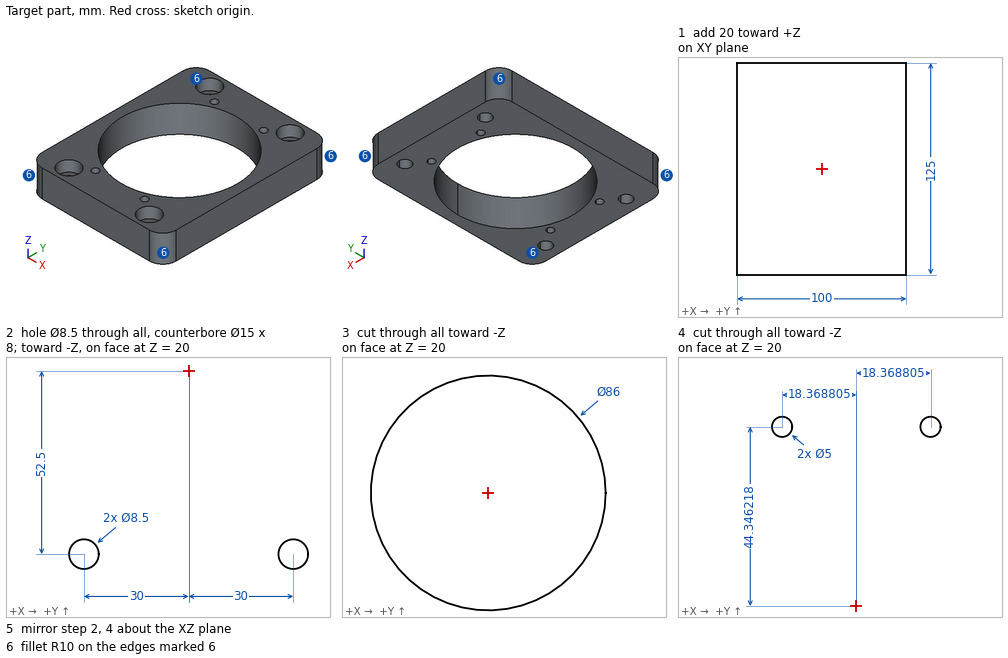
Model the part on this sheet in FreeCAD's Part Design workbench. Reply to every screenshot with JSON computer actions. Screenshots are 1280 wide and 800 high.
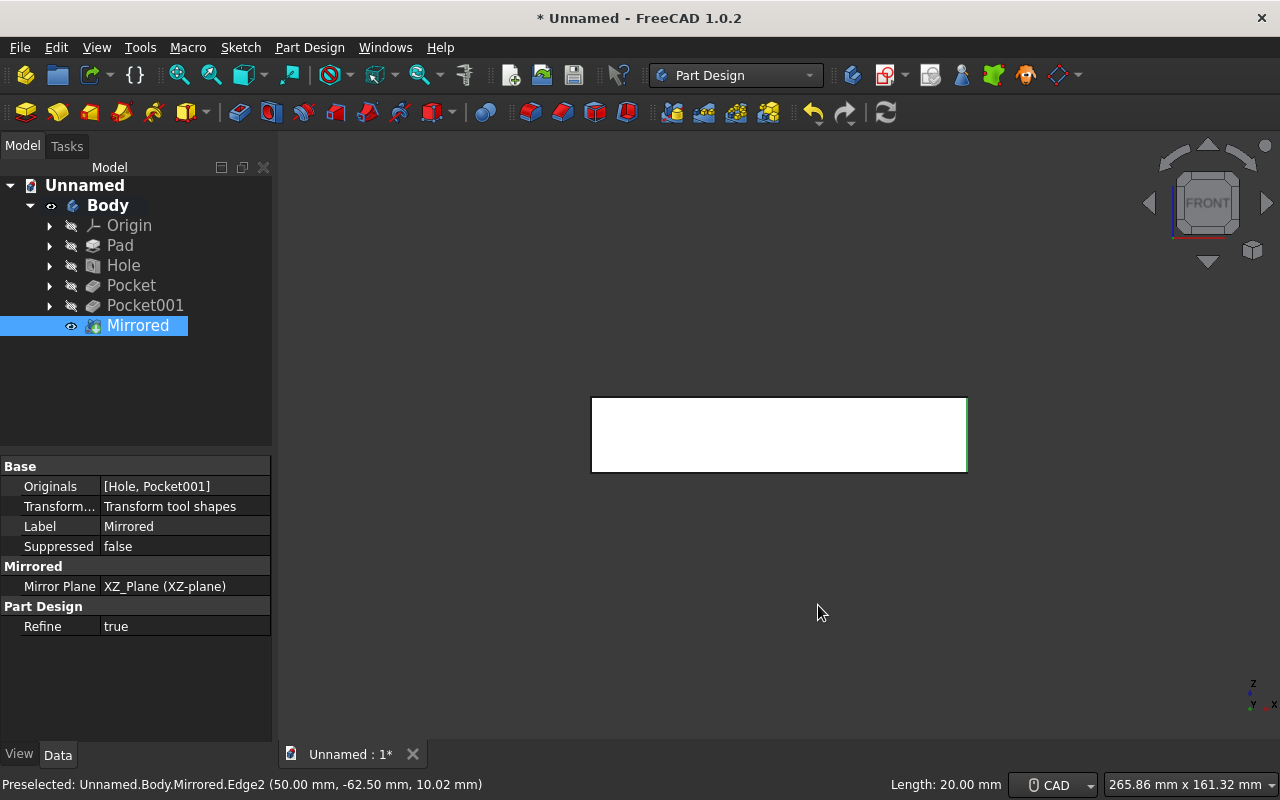
{"action": "left_click", "coordinate": [180, 76]}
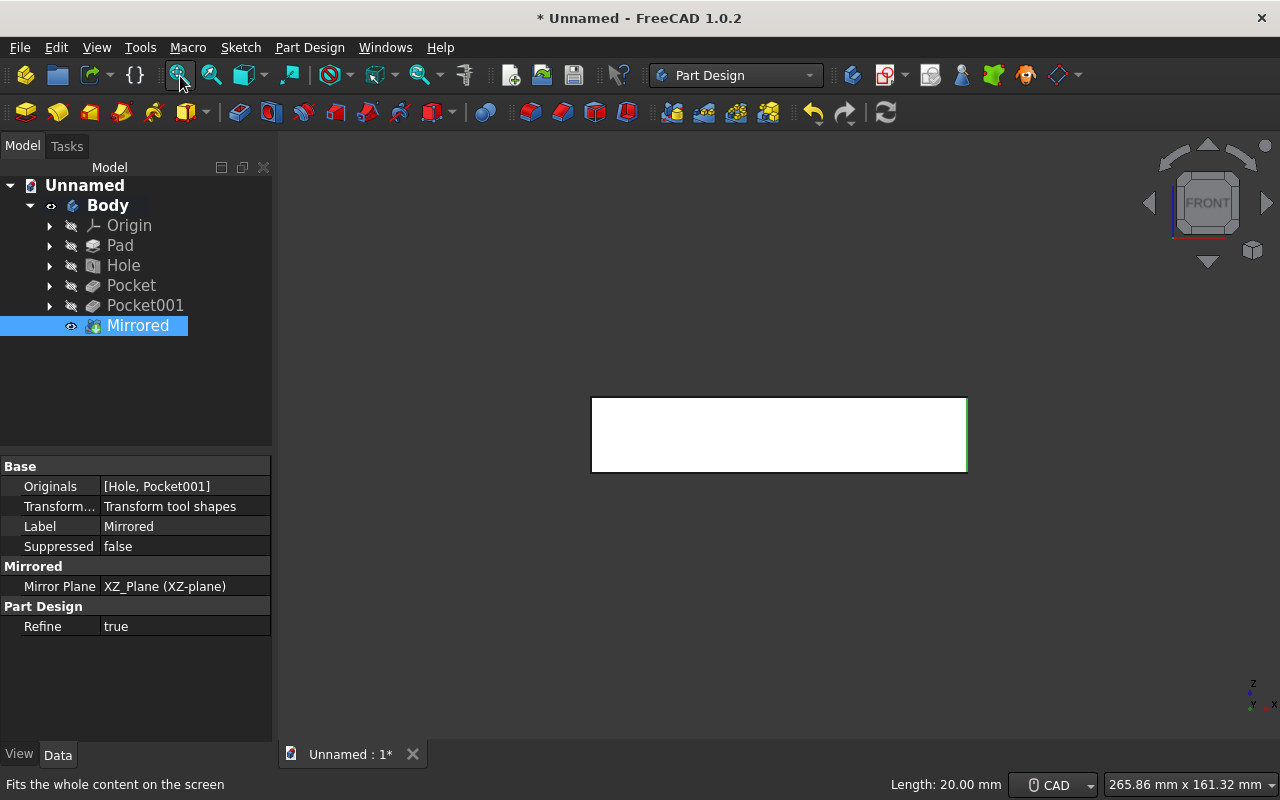
{"action": "left_click", "coordinate": [591, 434], "text": "ctrl"}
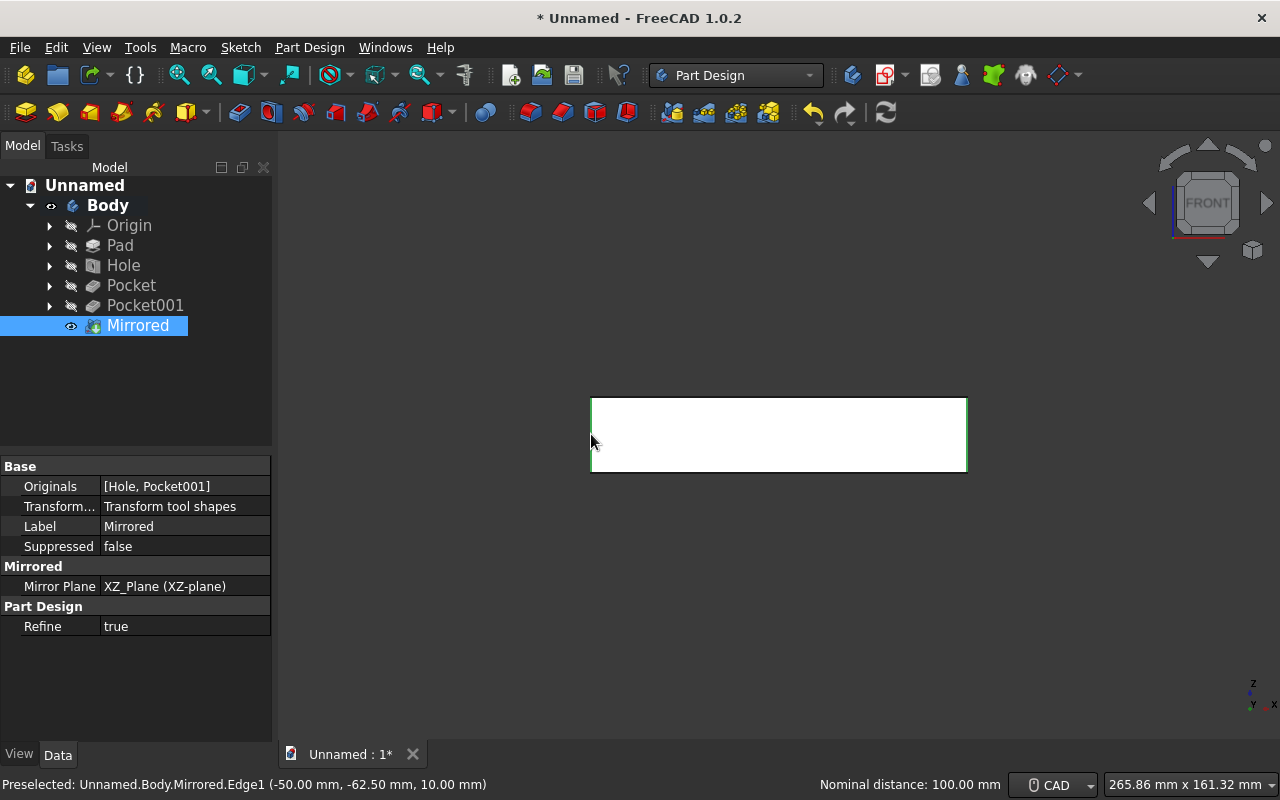
{"action": "key", "text": "3"}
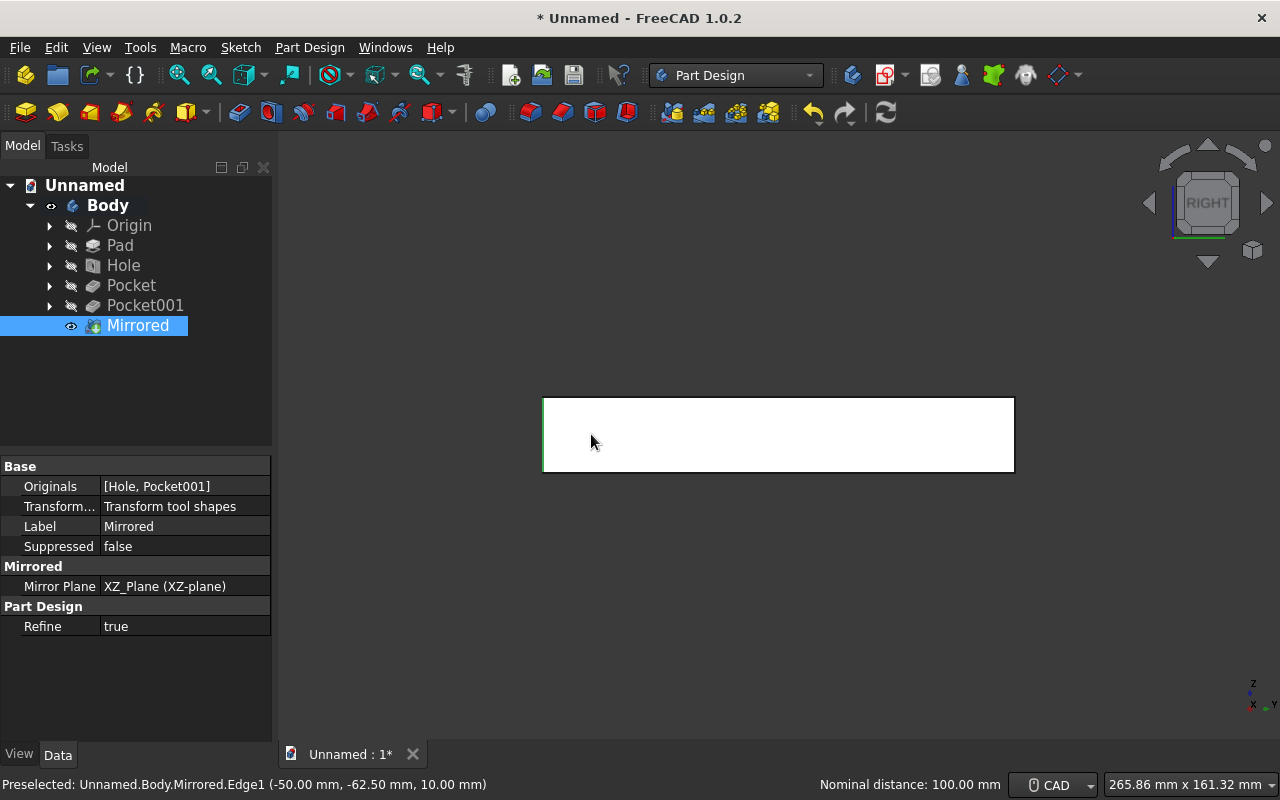
{"action": "left_click", "coordinate": [1015, 434], "text": "ctrl"}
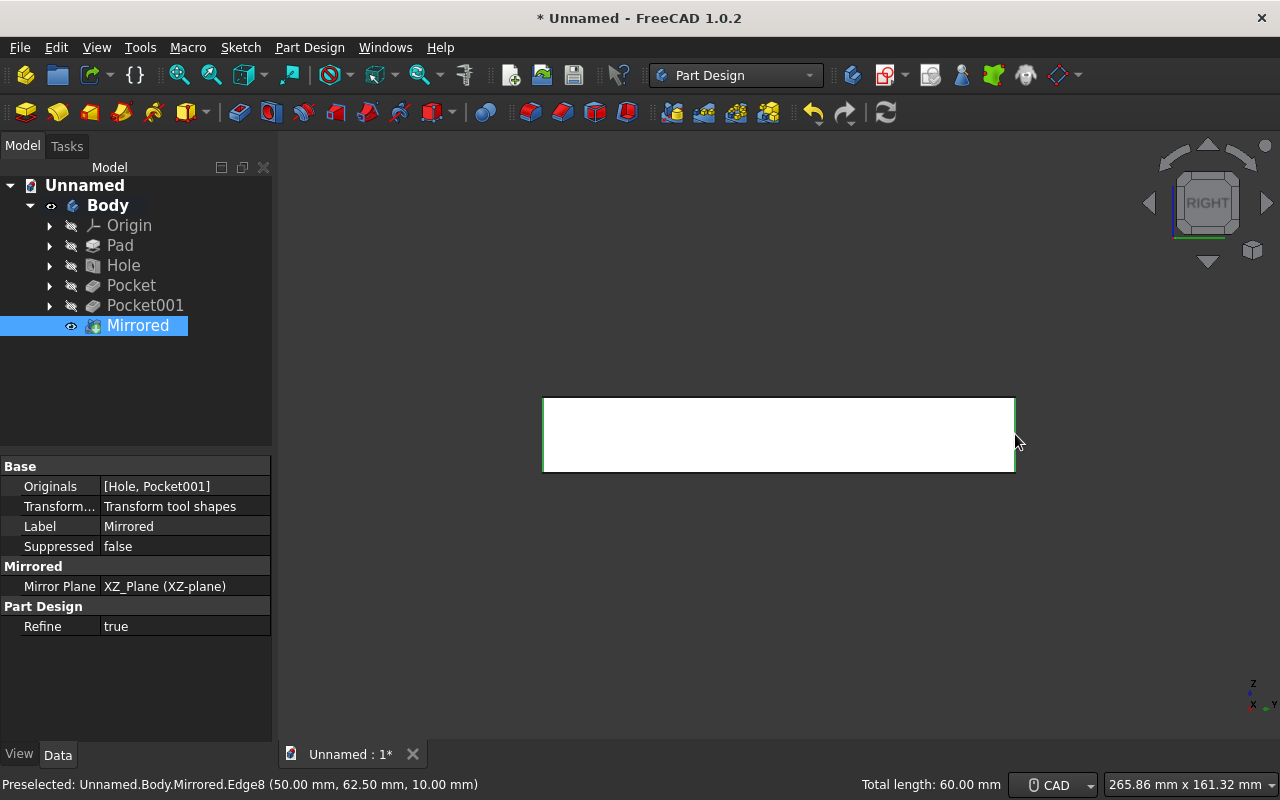
{"action": "key", "text": "5"}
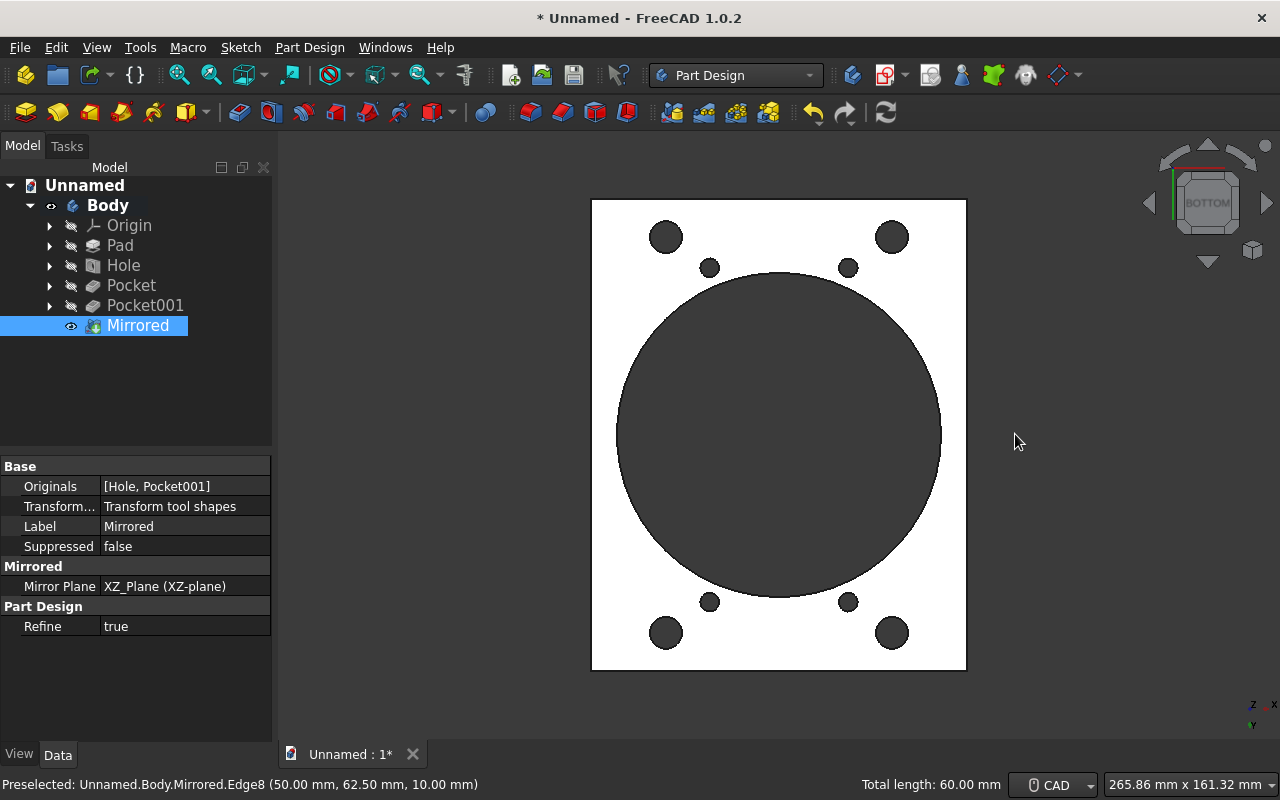
{"action": "key", "text": "4"}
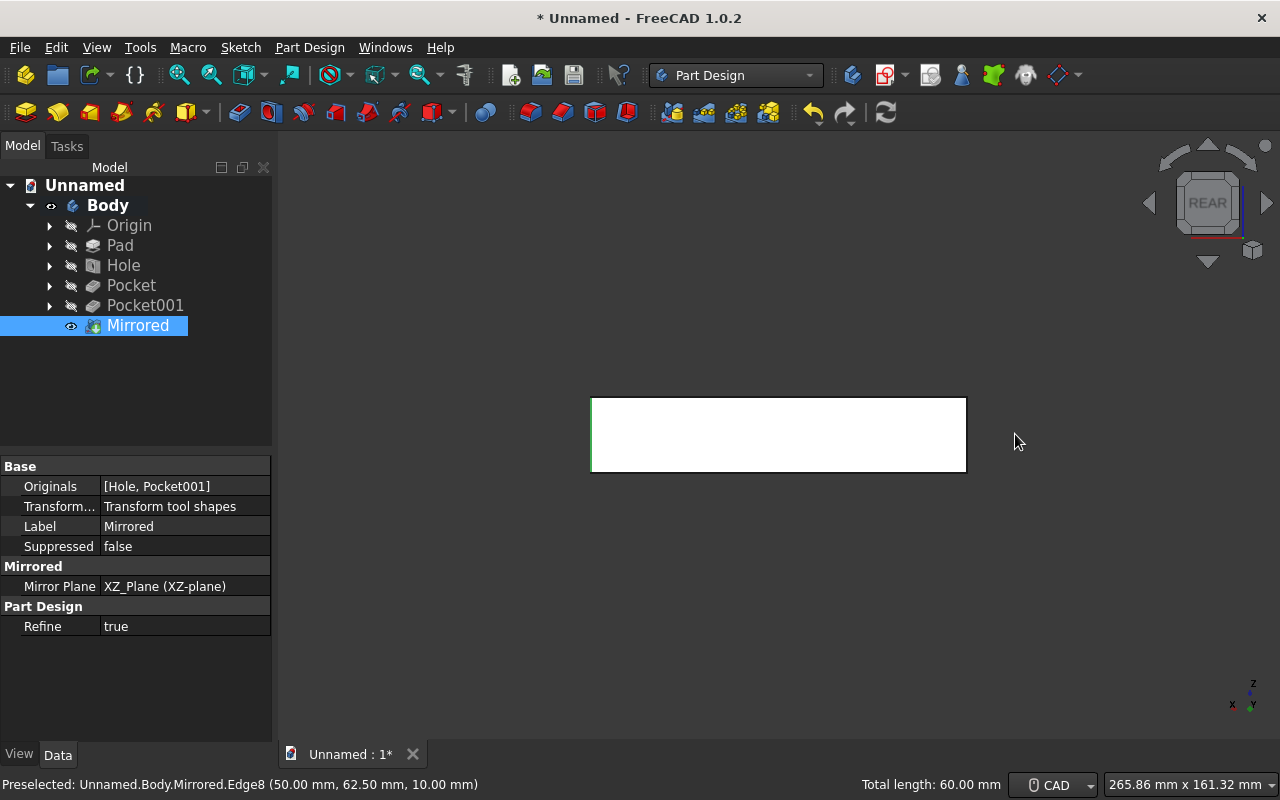
{"action": "left_click", "coordinate": [180, 76]}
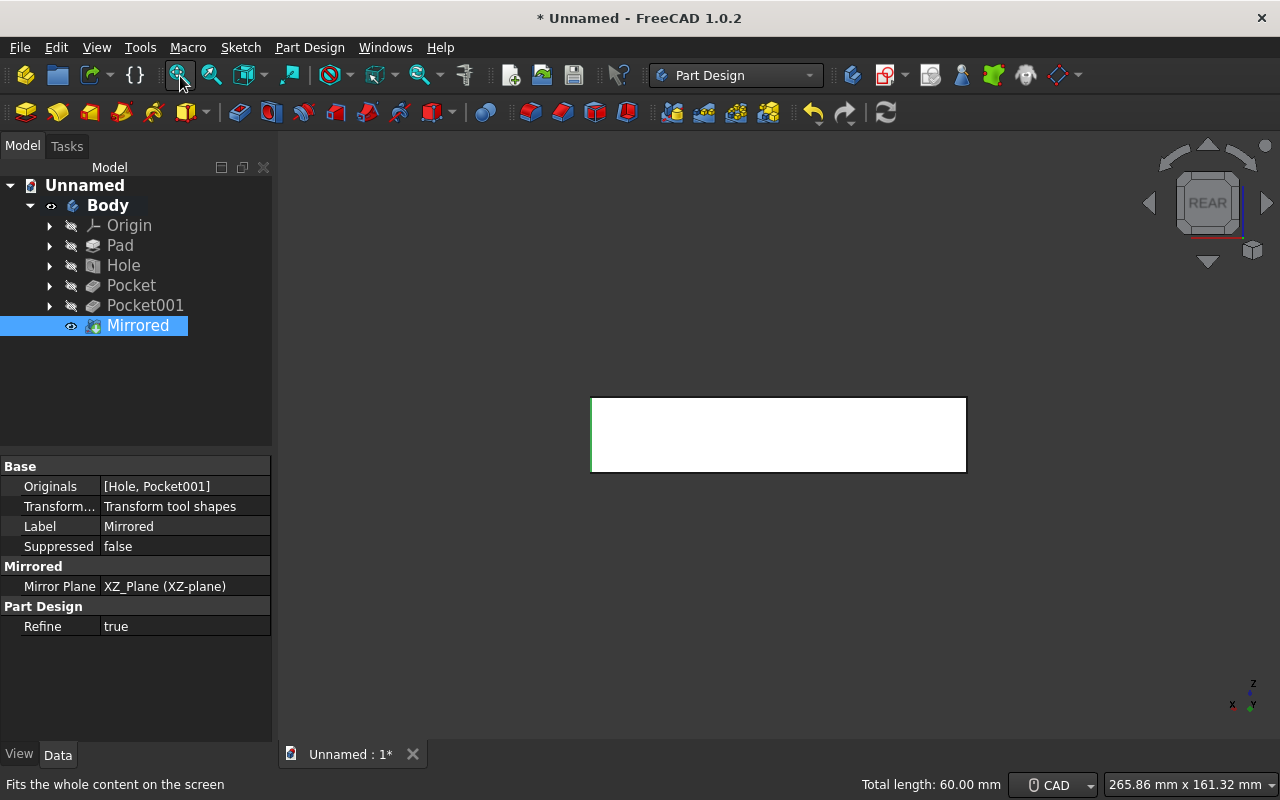
{"action": "left_click", "coordinate": [967, 434], "text": "ctrl"}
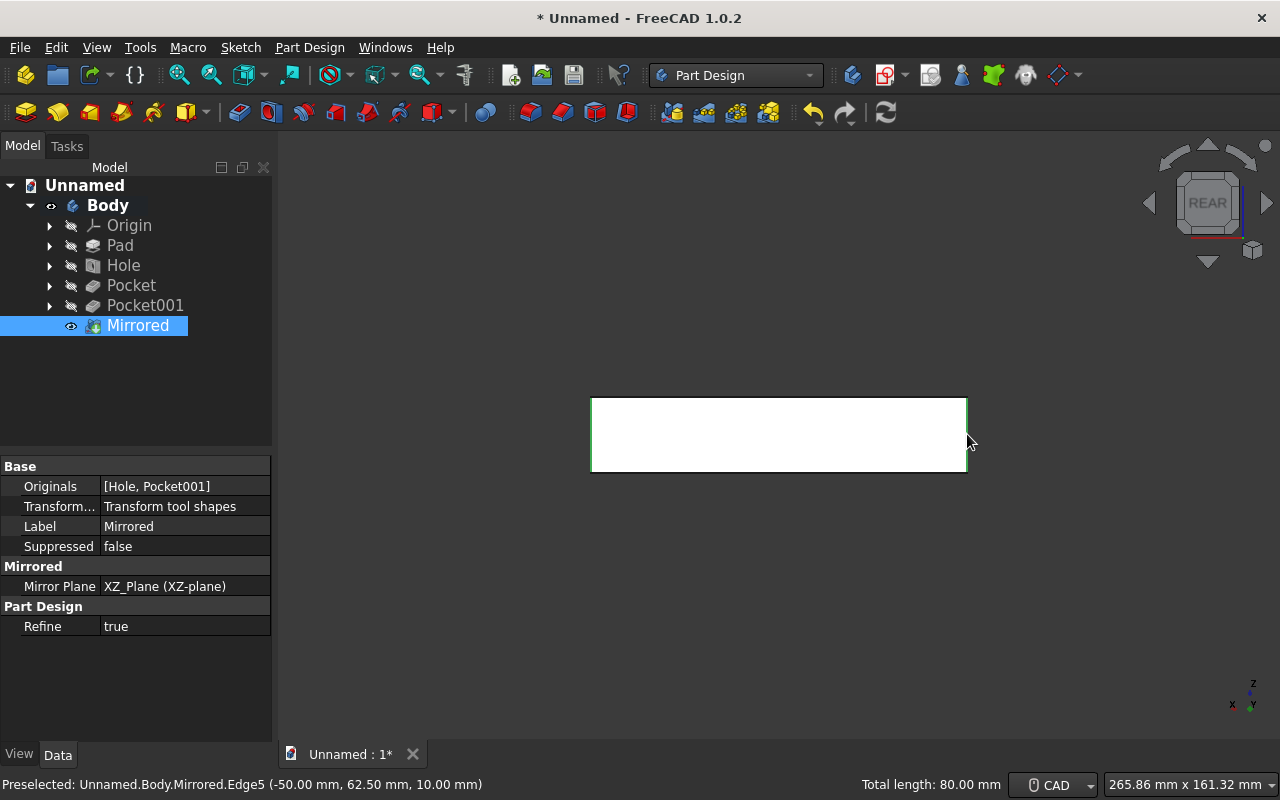
{"action": "left_click", "coordinate": [532, 112]}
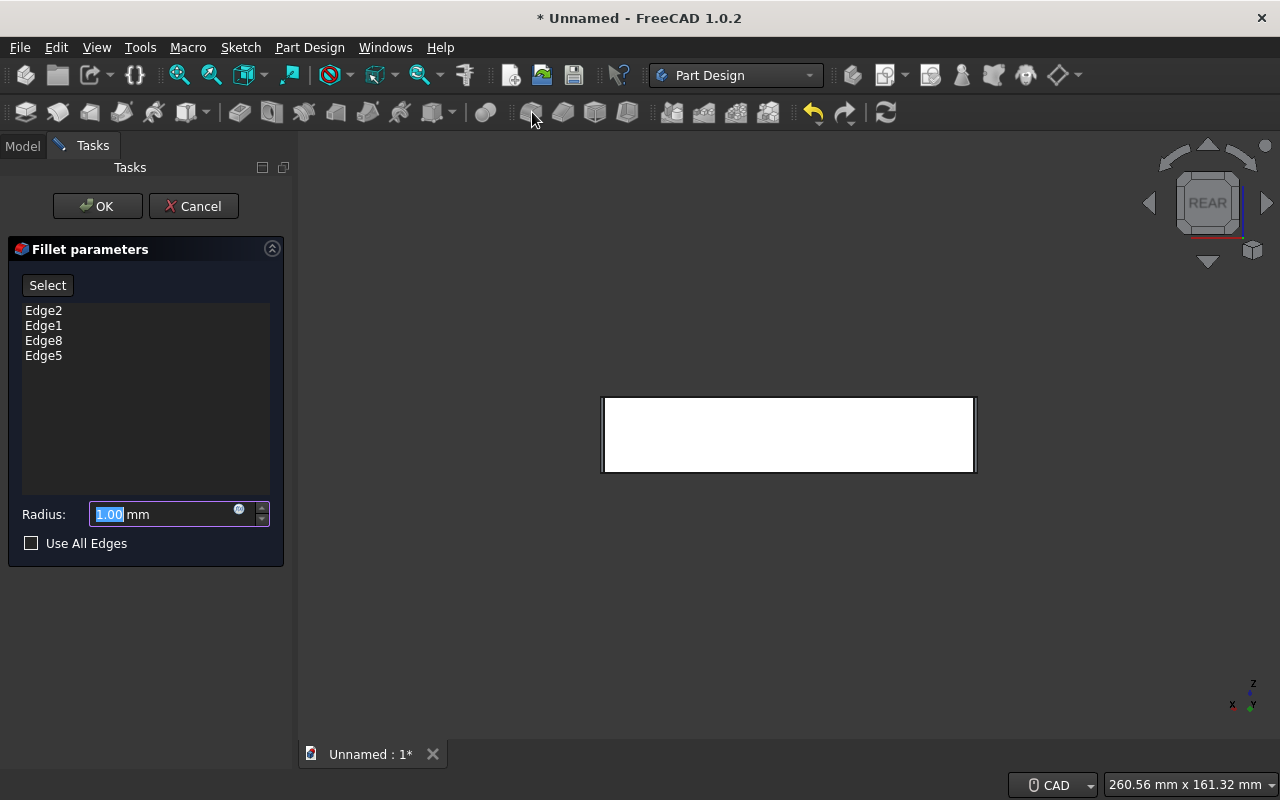
{"action": "type", "text": "10"}
{"action": "key", "text": "Tab"}